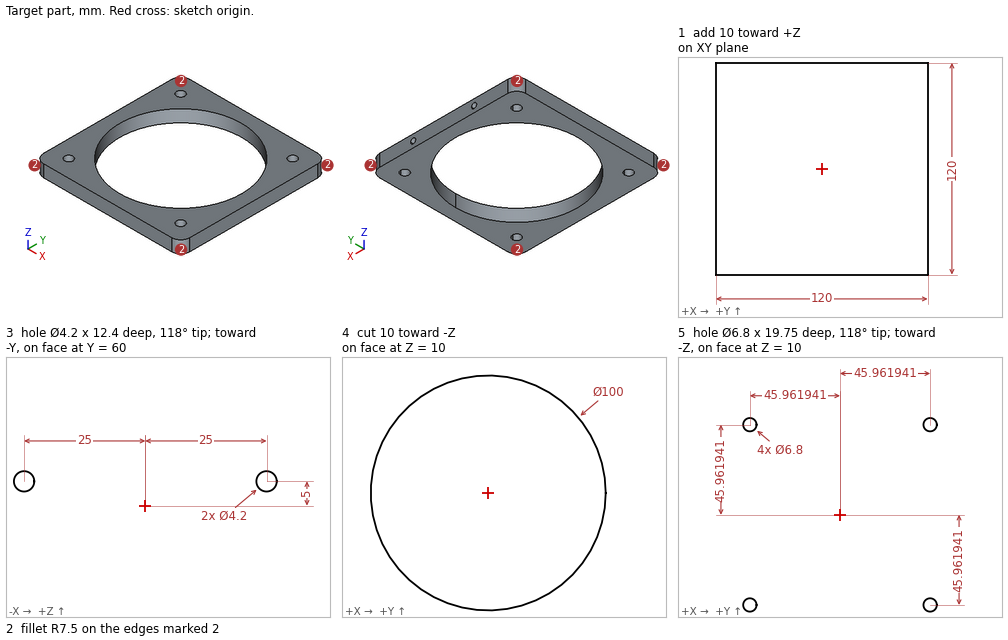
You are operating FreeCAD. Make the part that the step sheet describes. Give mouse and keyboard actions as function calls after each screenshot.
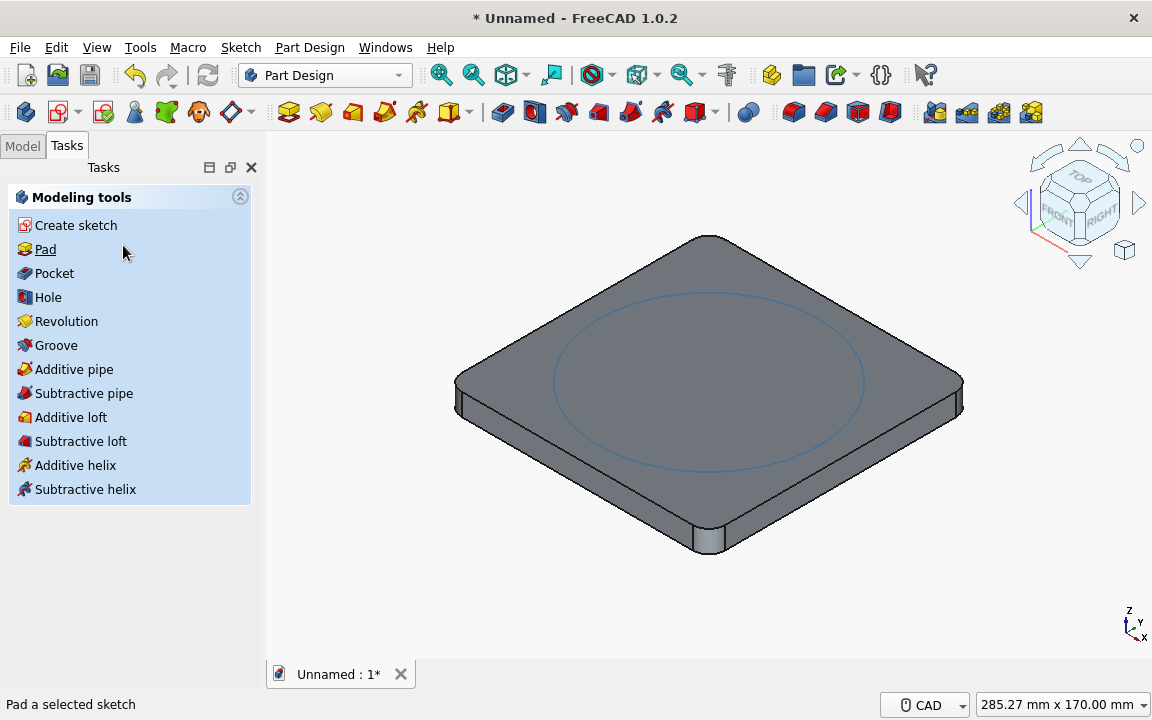
click(504, 112)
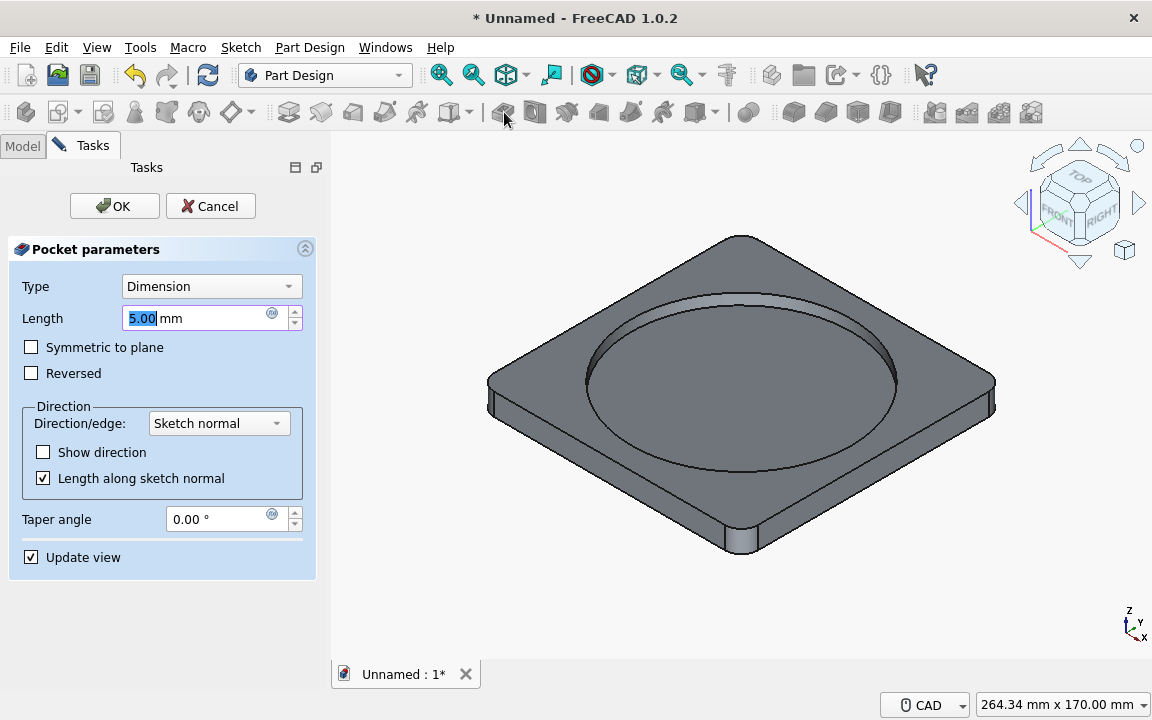
text(10)
key(Tab)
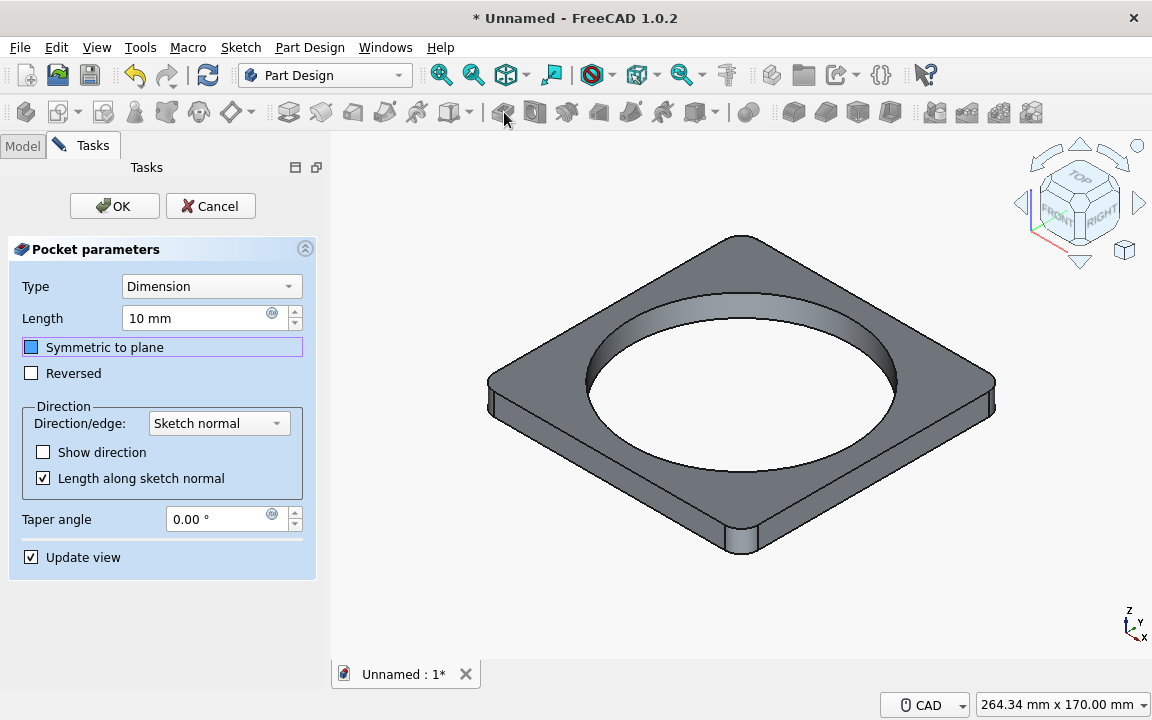
click(115, 206)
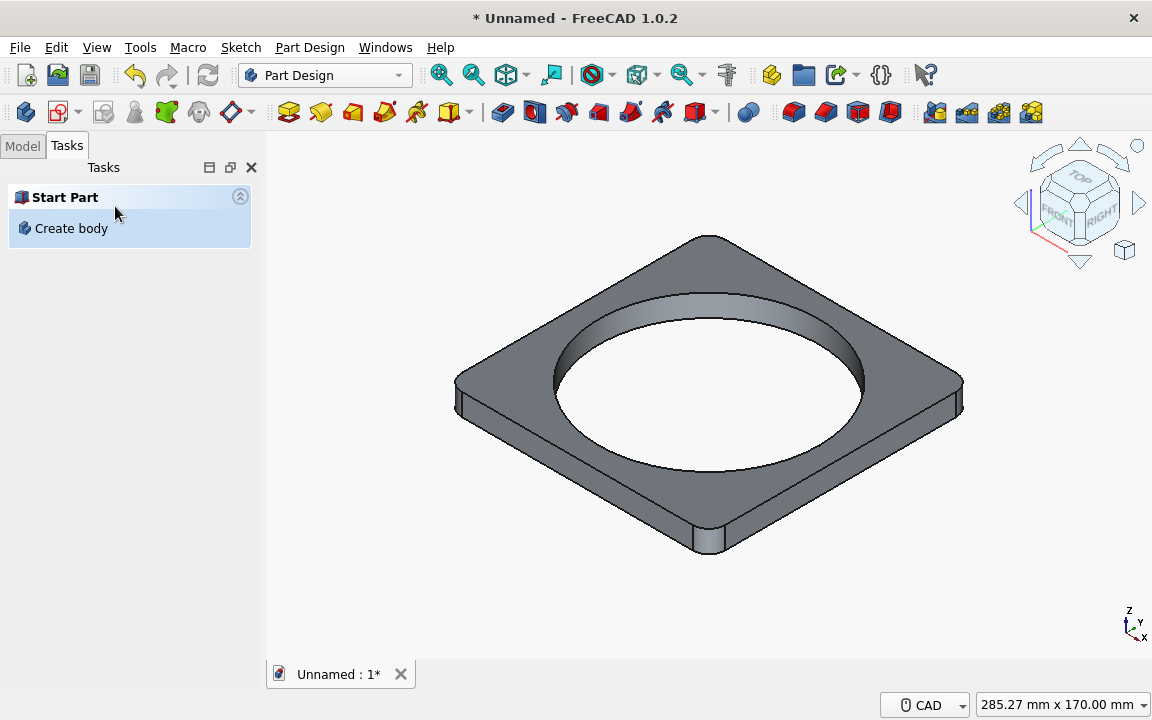
click(935, 381)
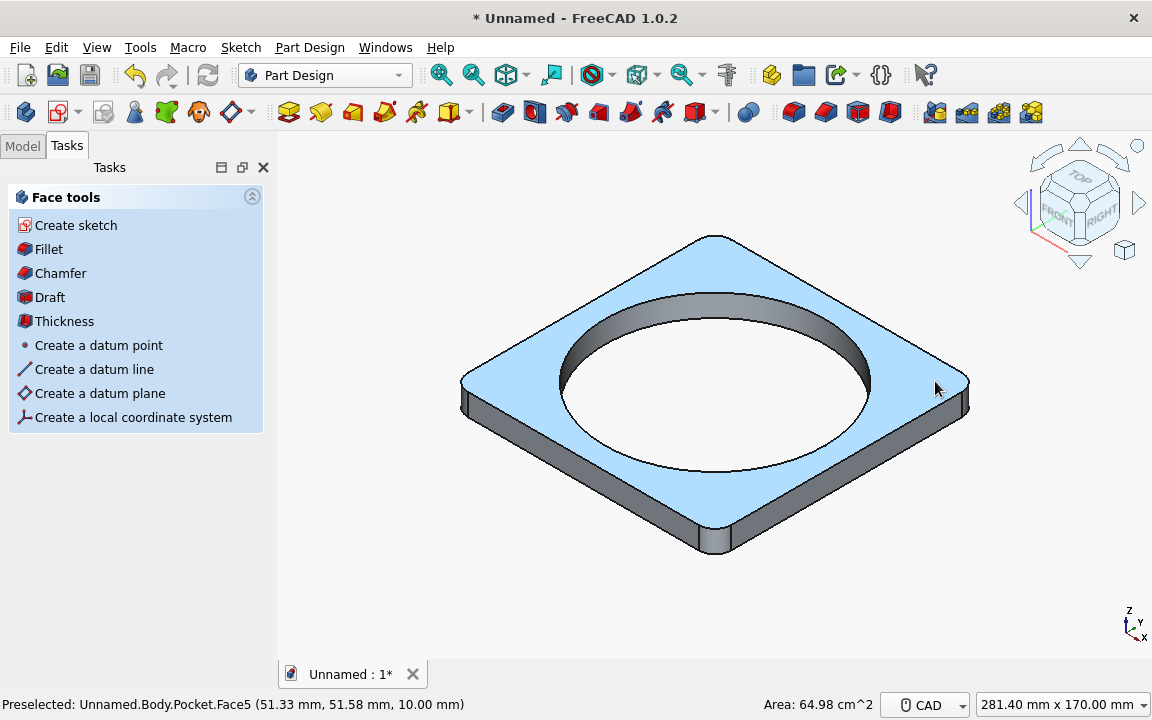
click(58, 112)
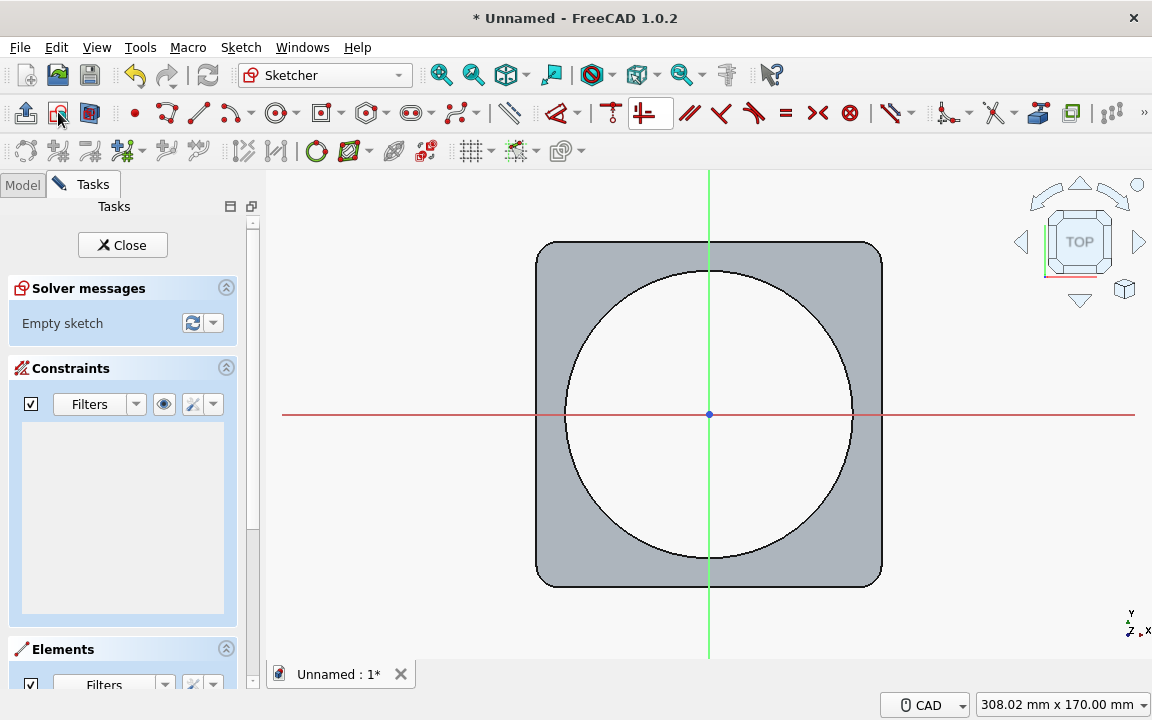
click(276, 114)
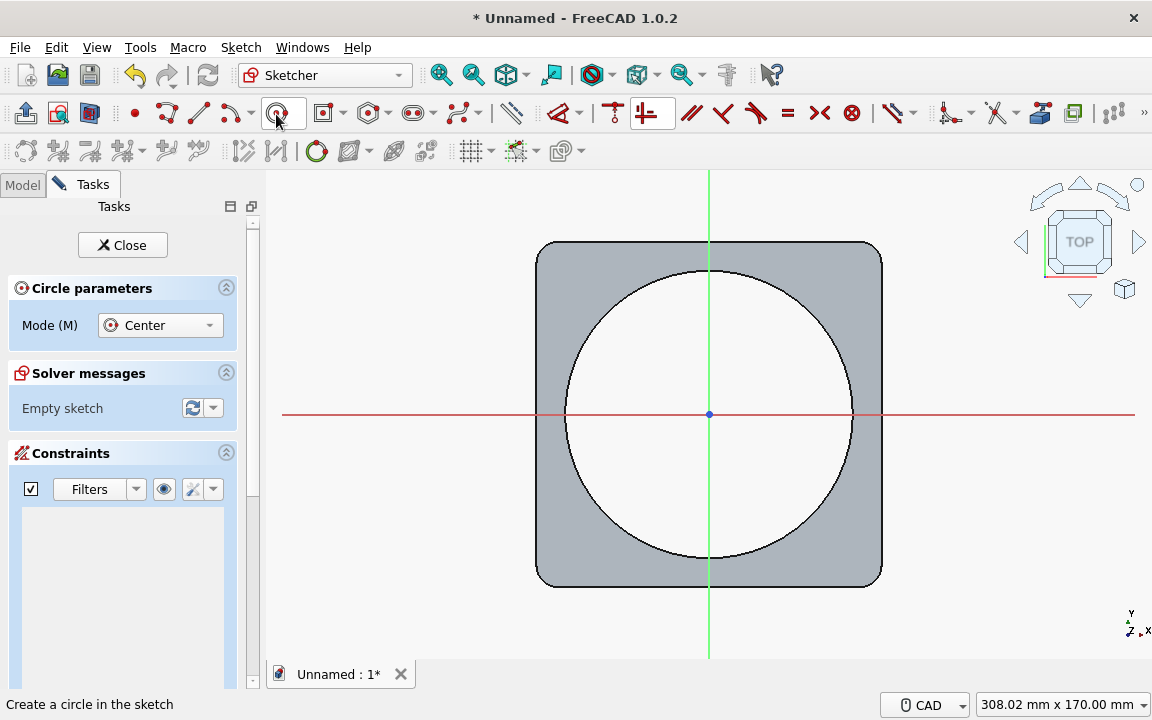
scroll(577, 282, up, 5)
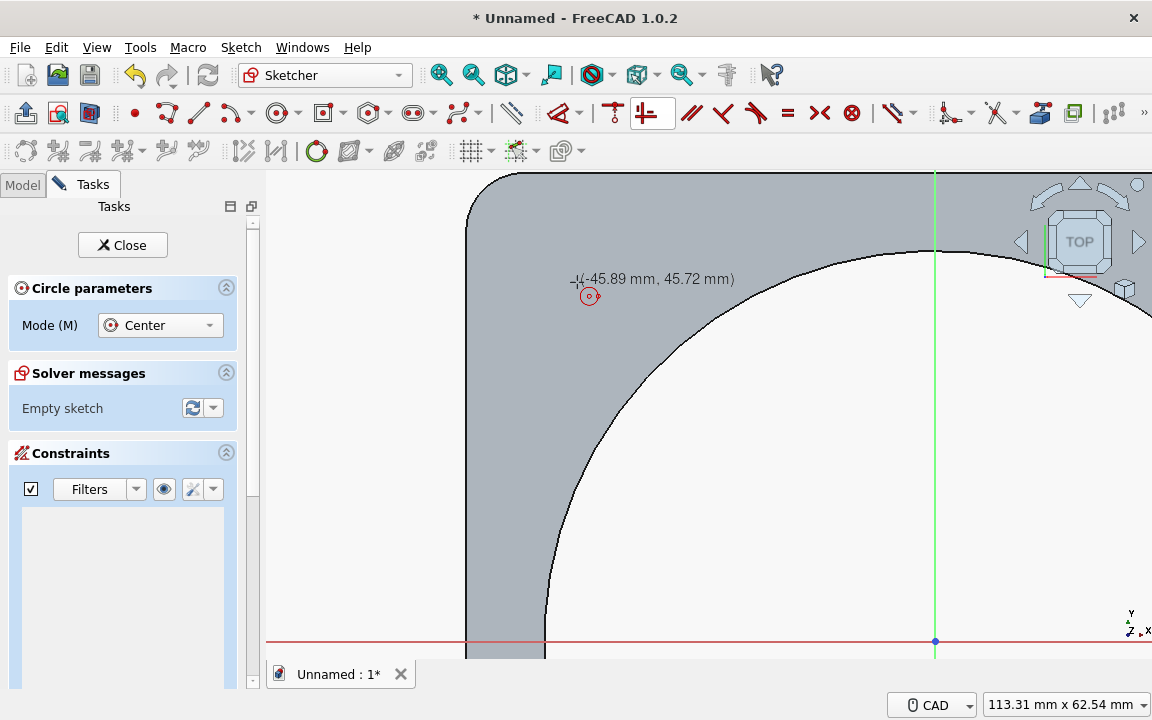
click(576, 282)
click(595, 264)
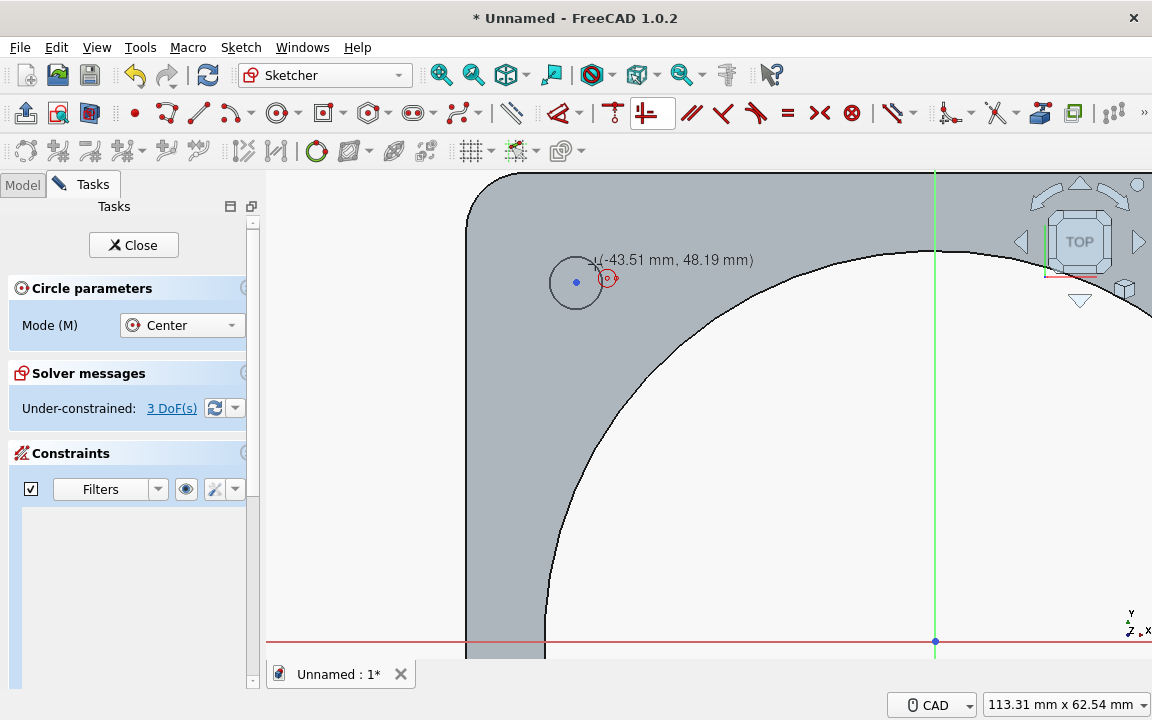
scroll(469, 282, down, 5)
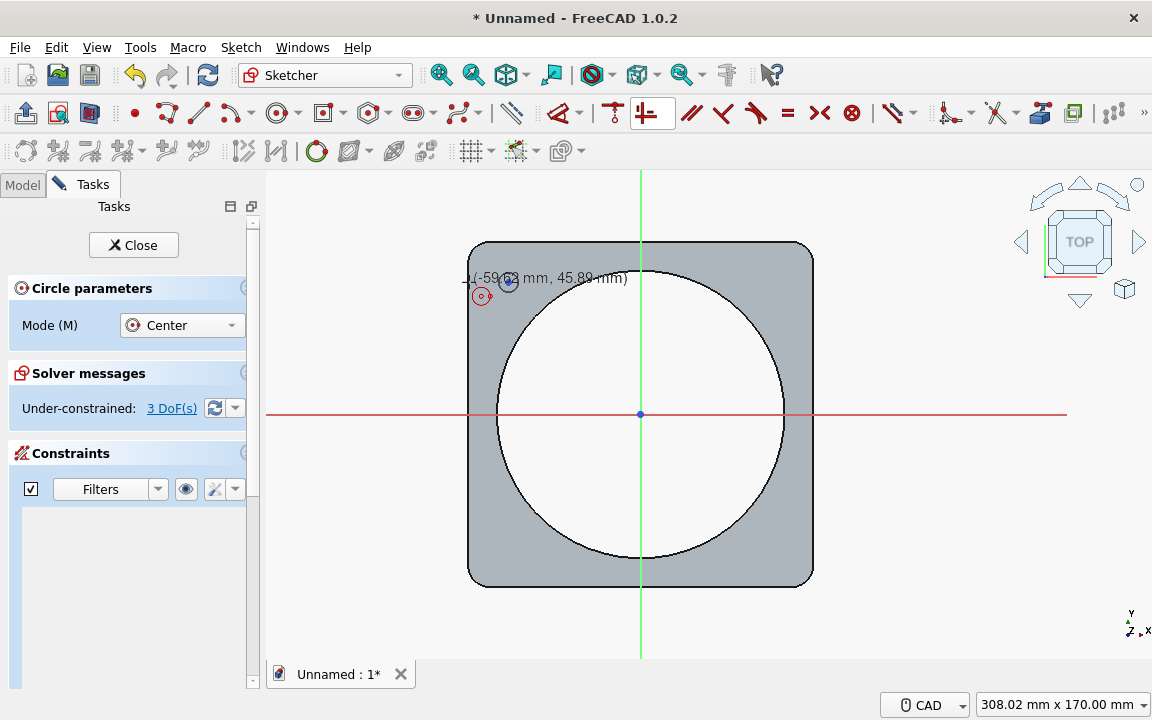
scroll(773, 282, up, 5)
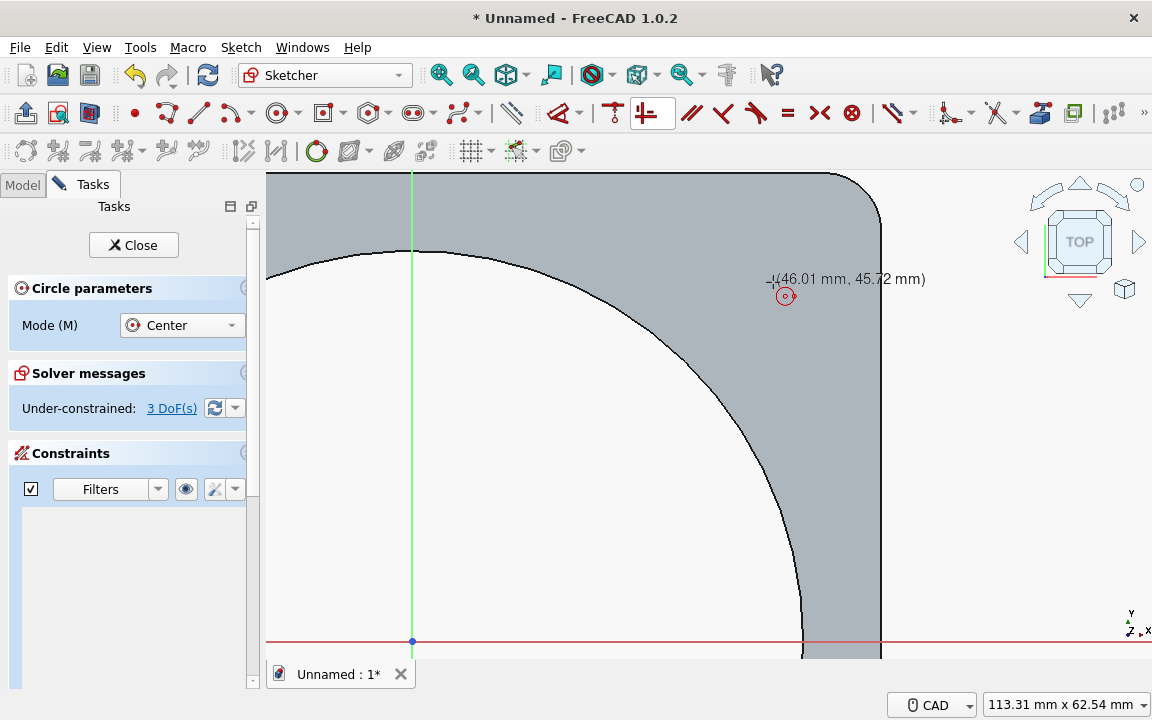
click(772, 282)
click(790, 264)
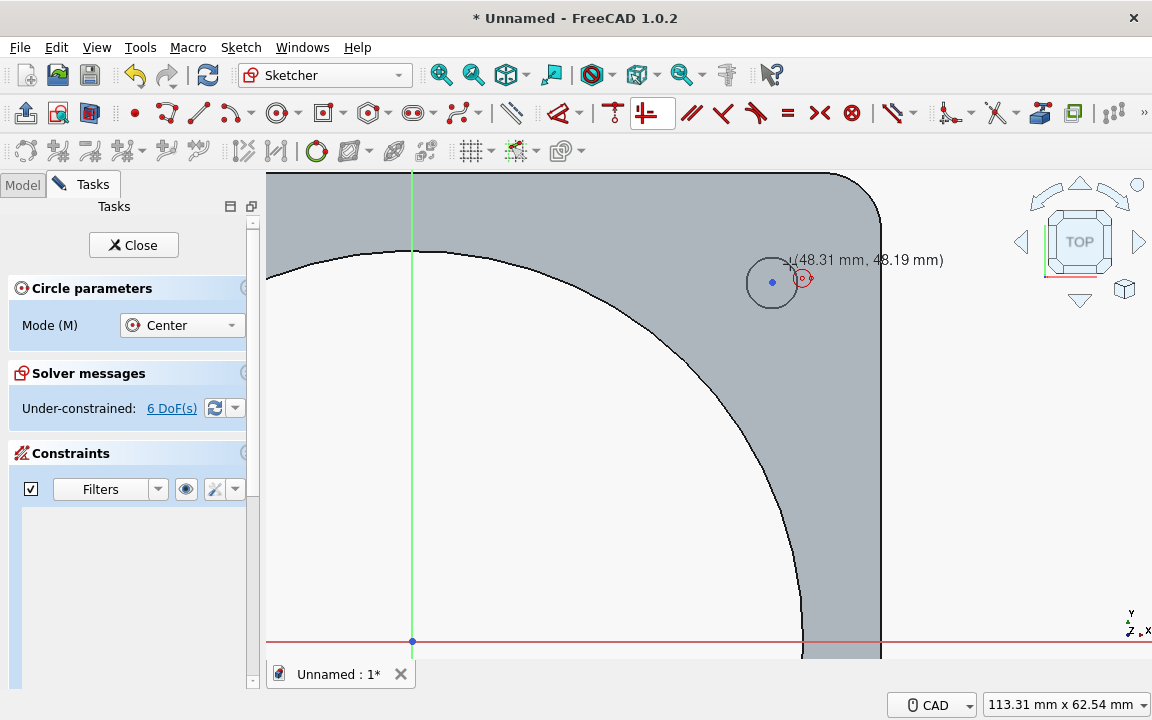
scroll(773, 282, down, 5)